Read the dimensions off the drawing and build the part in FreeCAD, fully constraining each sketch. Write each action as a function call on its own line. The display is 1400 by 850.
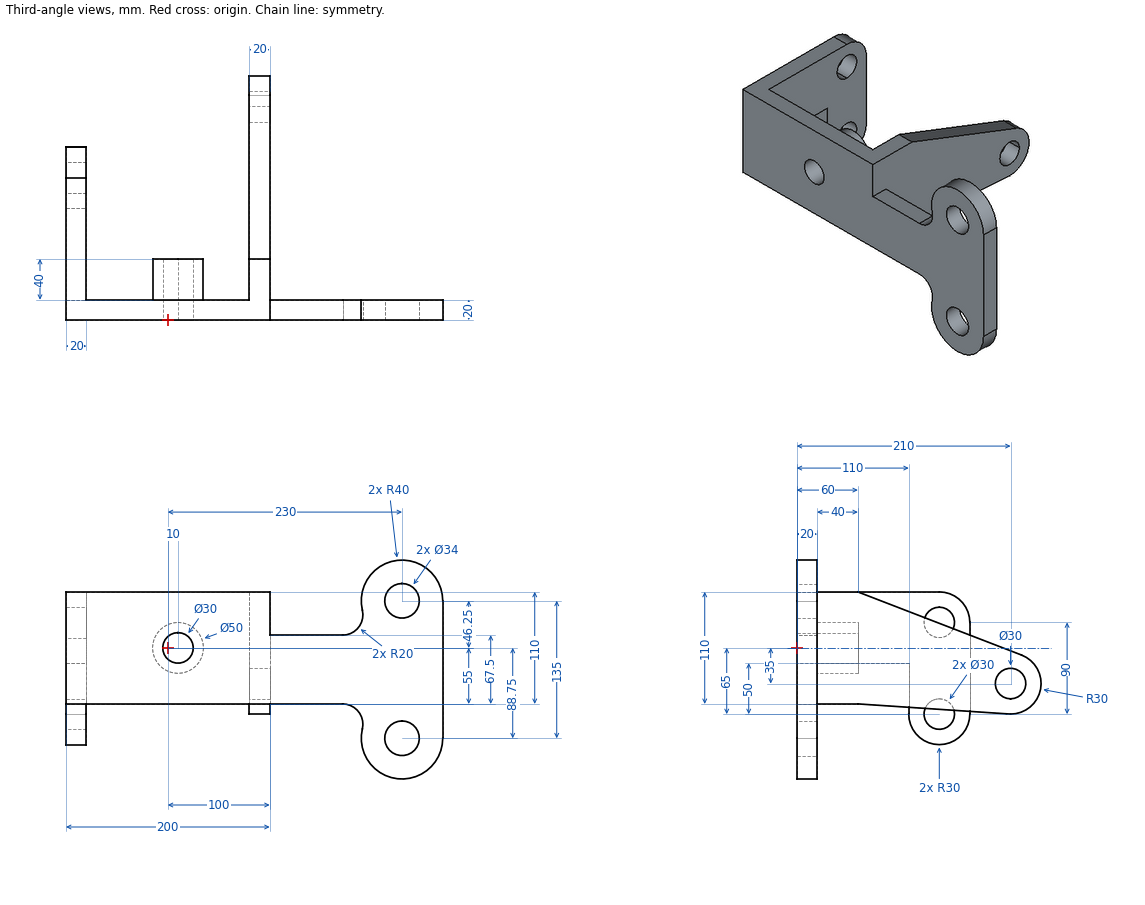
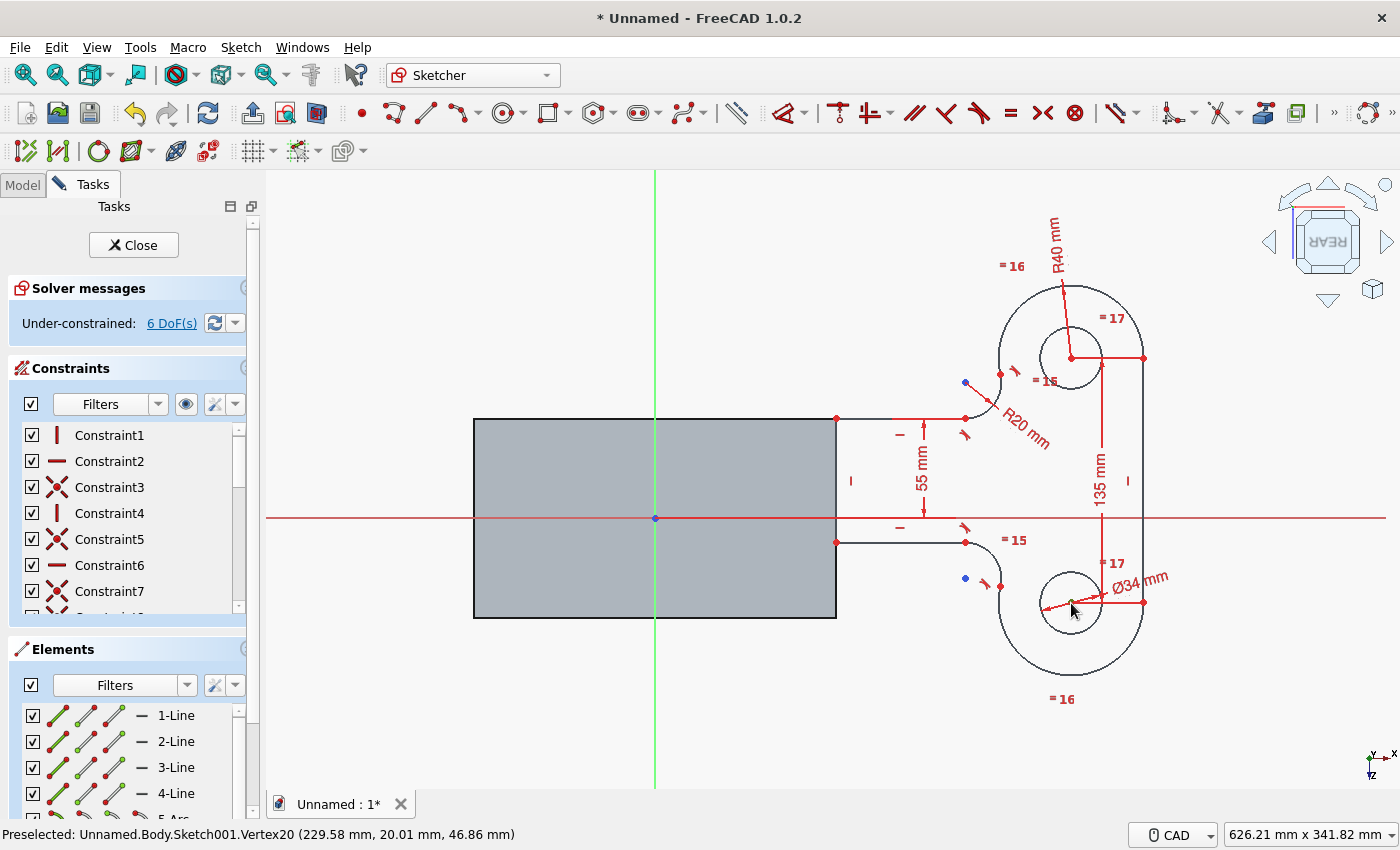
key(l)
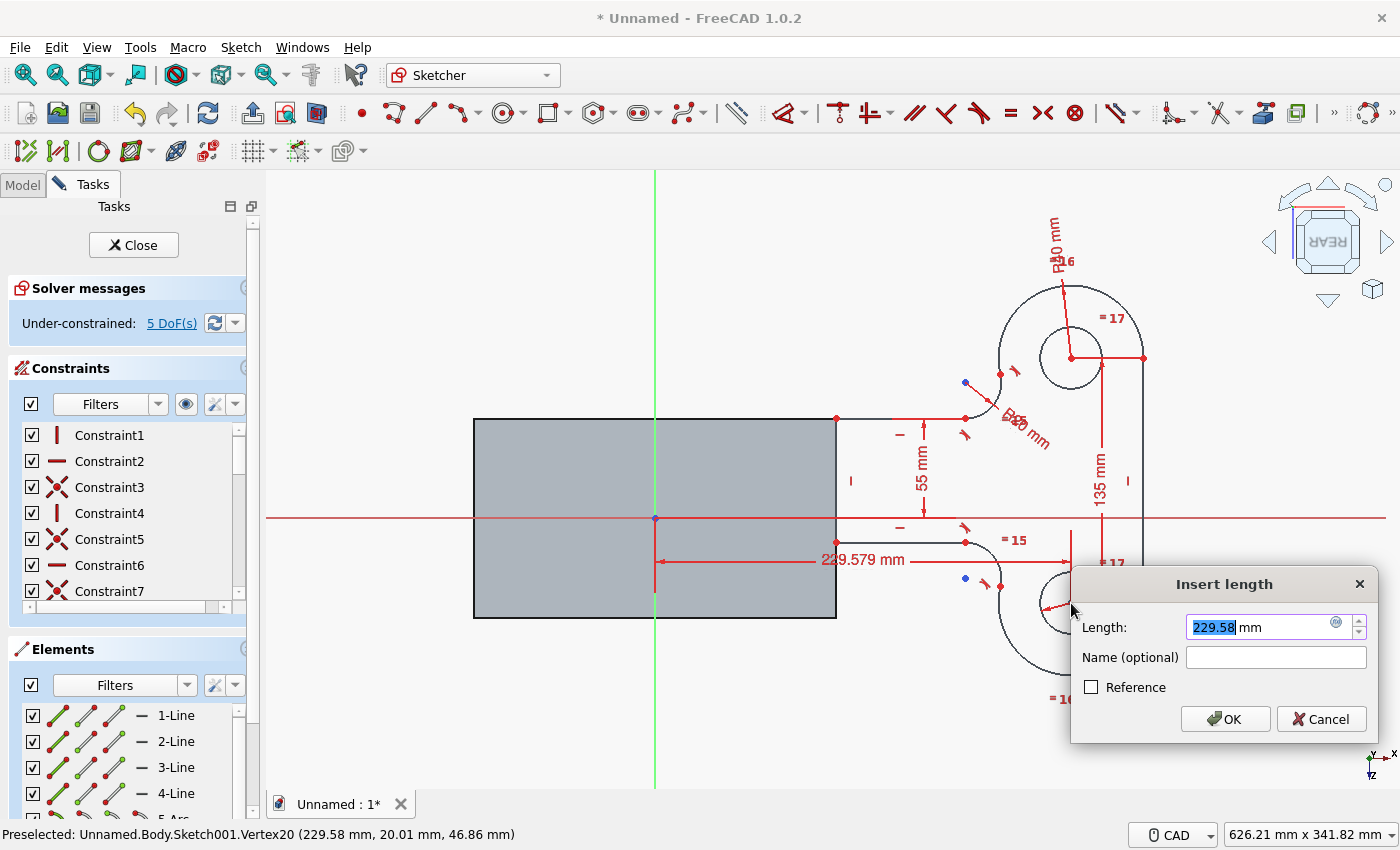
text(230)
key(Return)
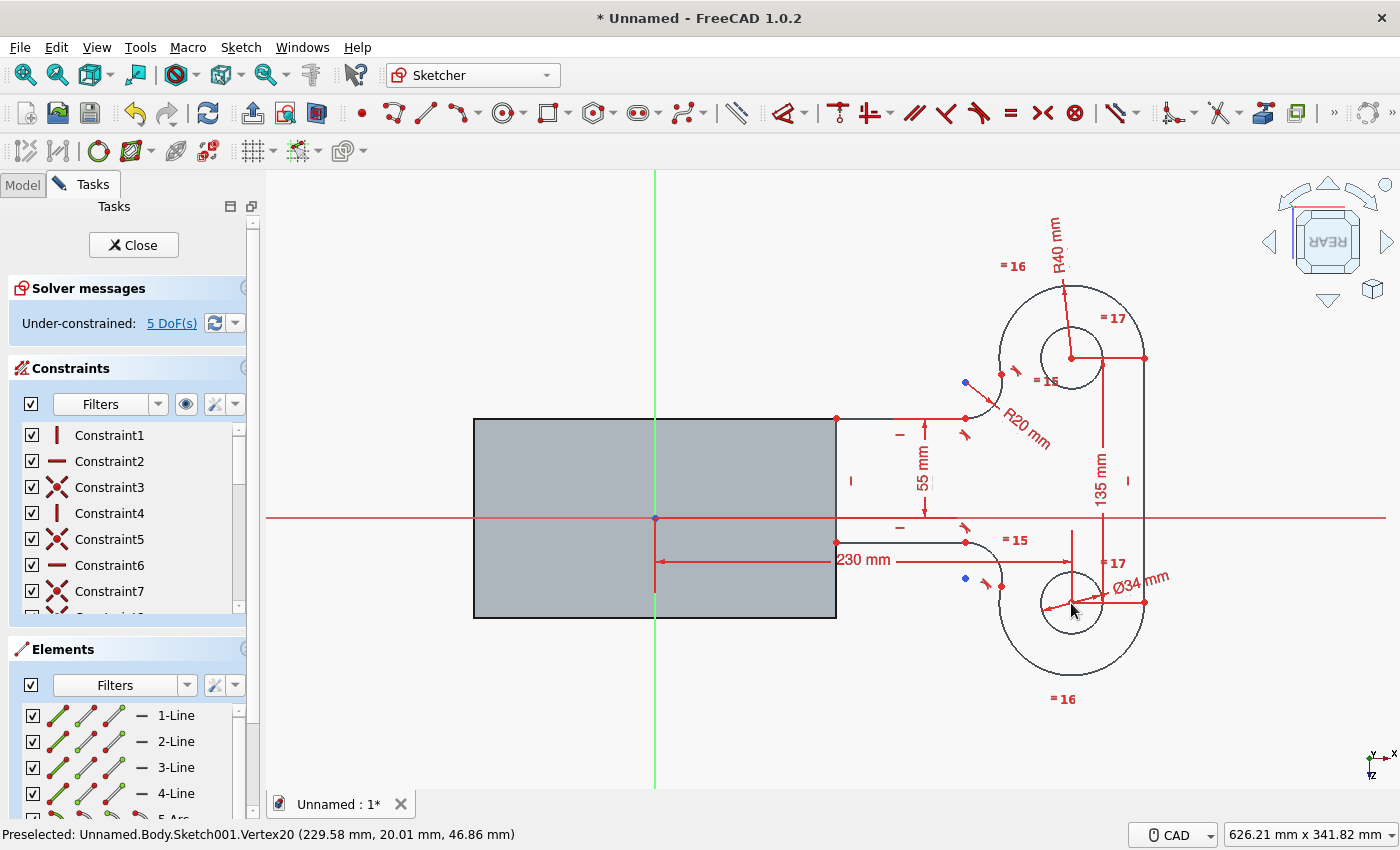
click(836, 456)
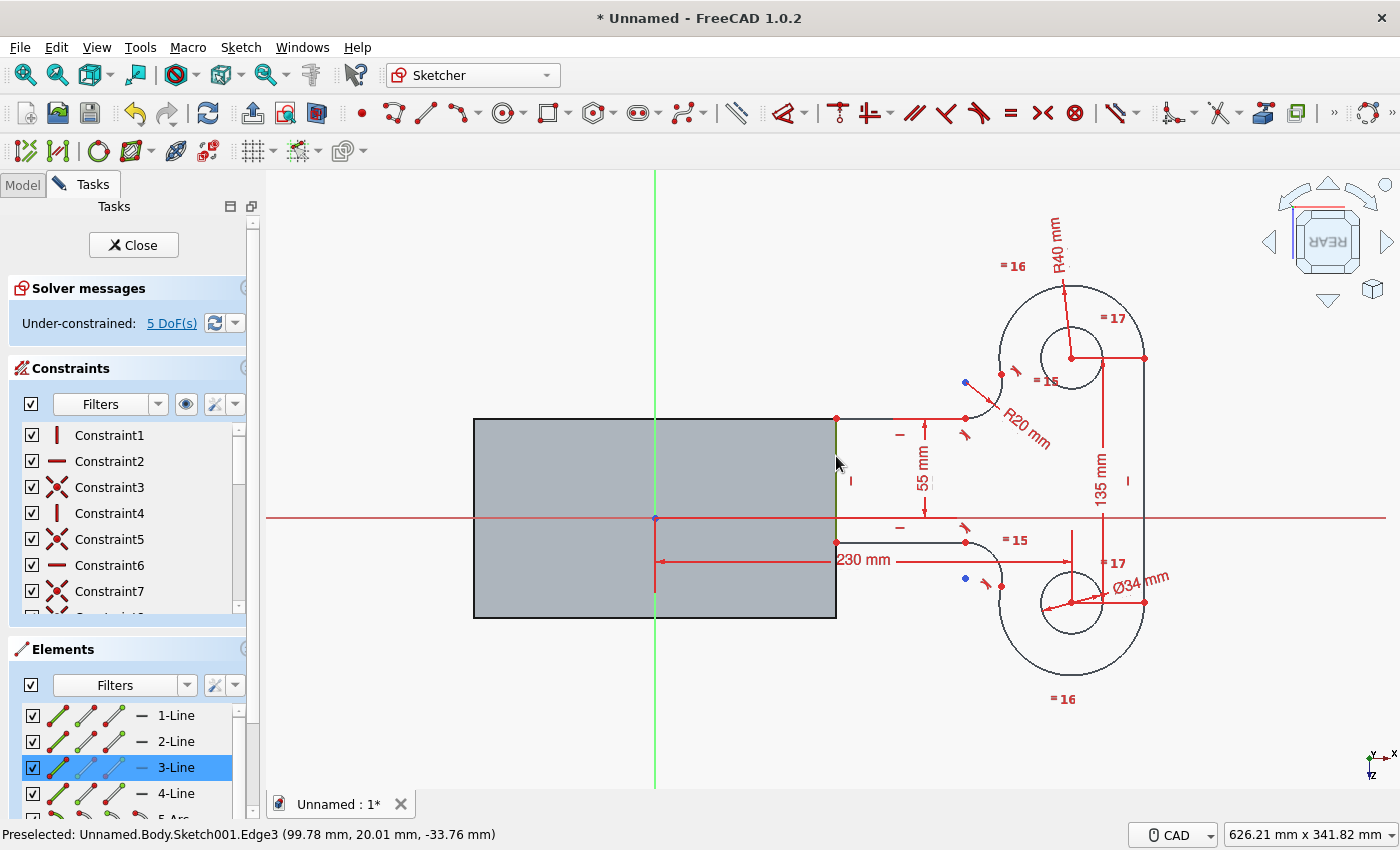
key(i)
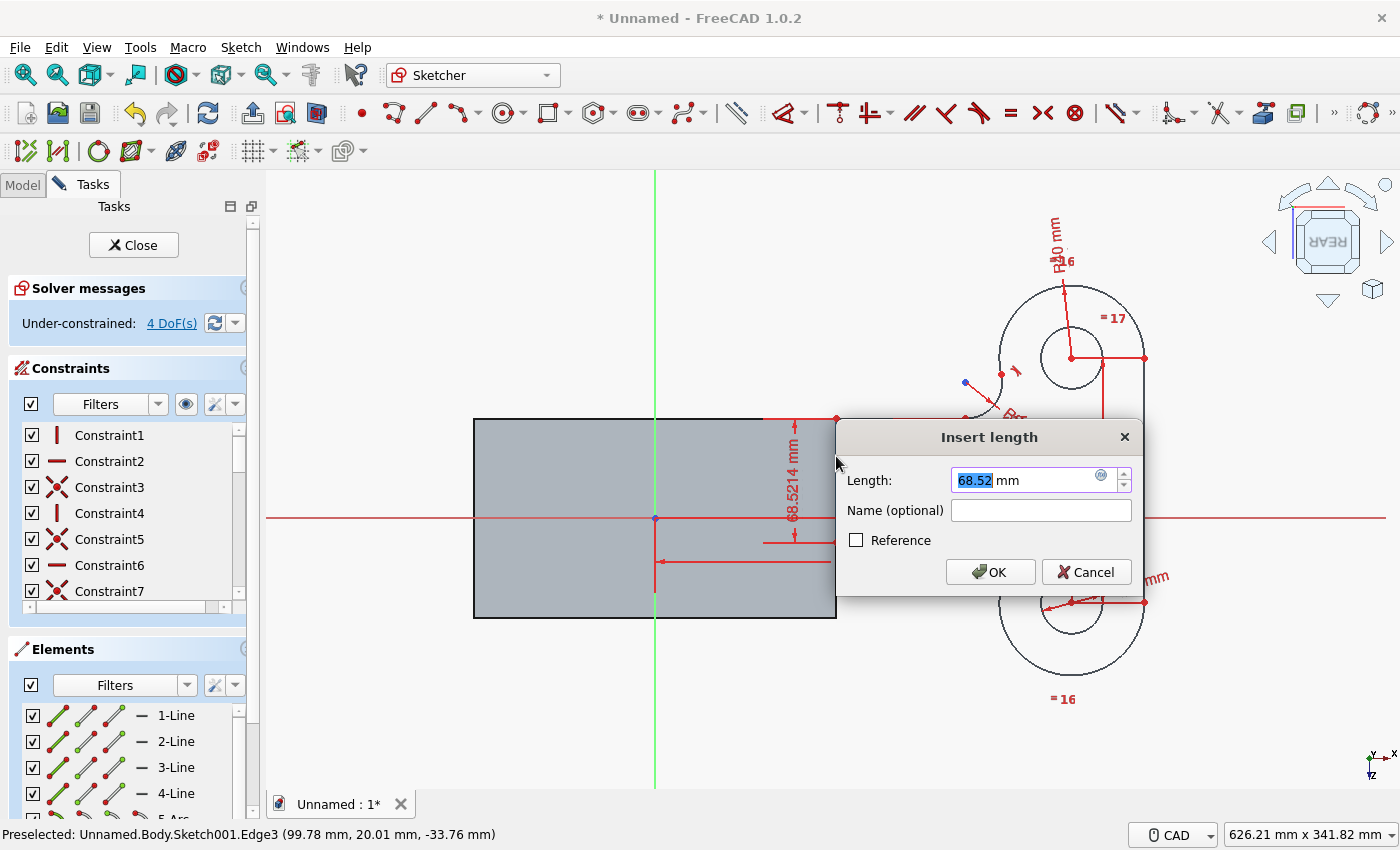
text(67.5)
key(Return)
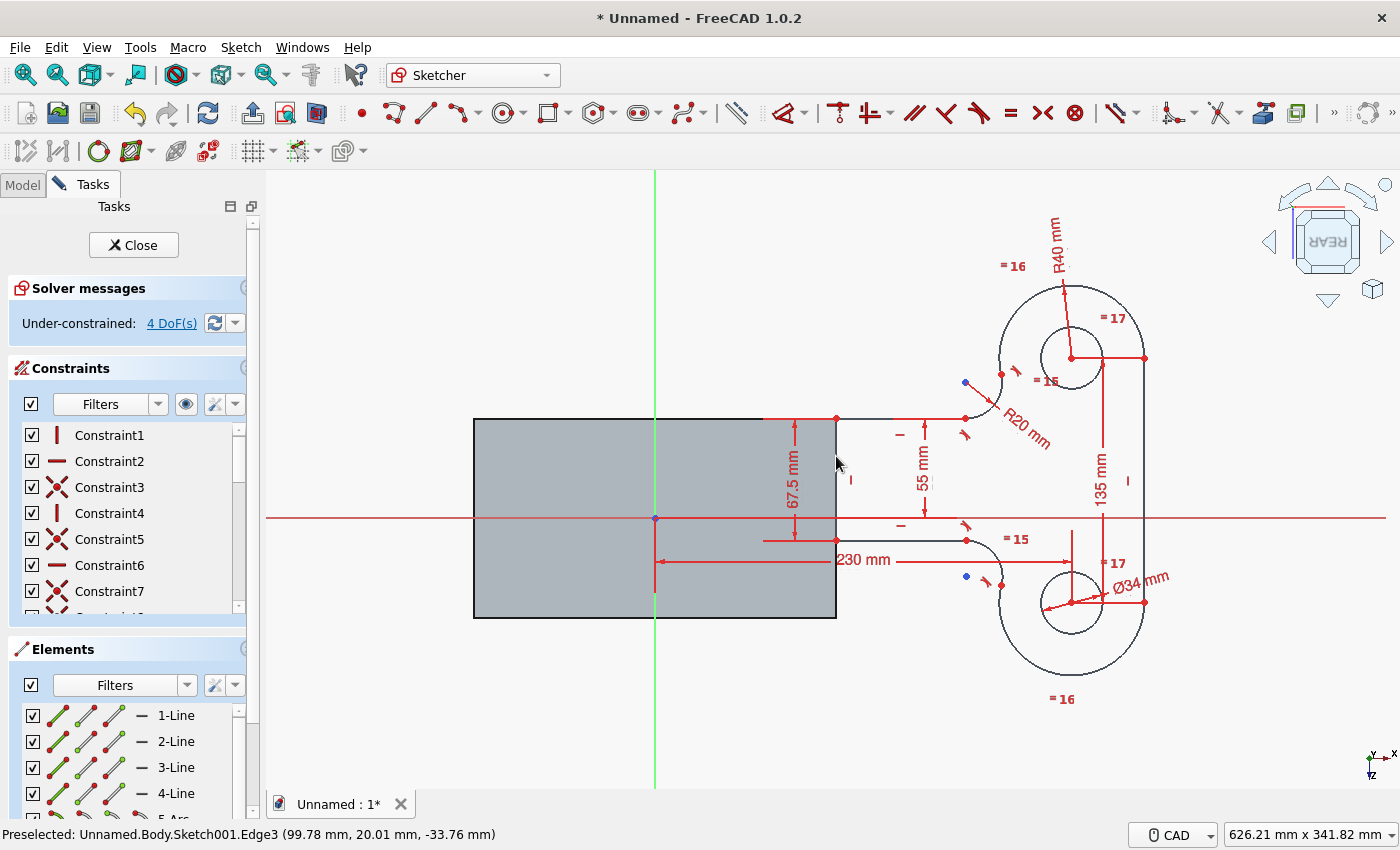
click(836, 419)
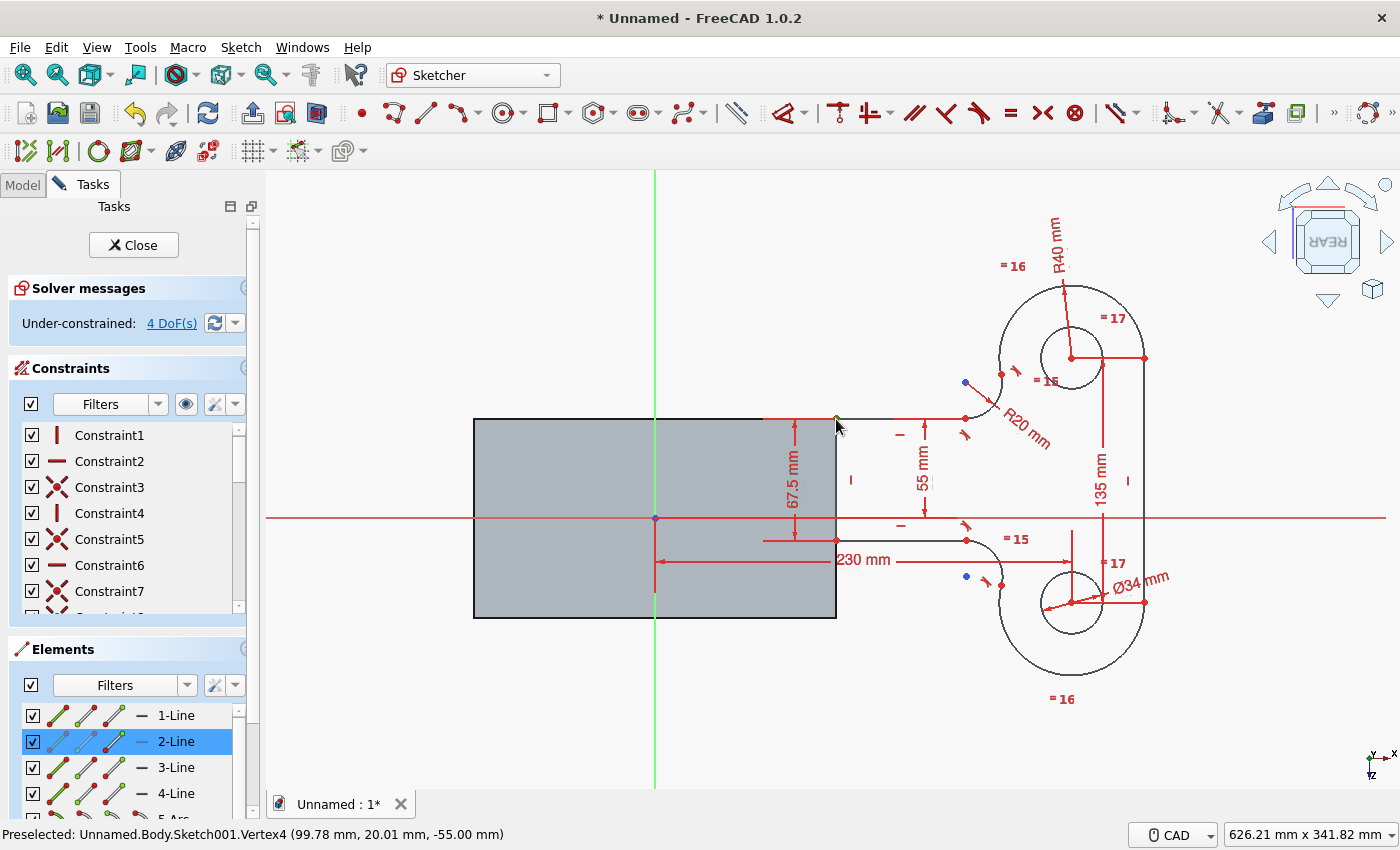
click(806, 114)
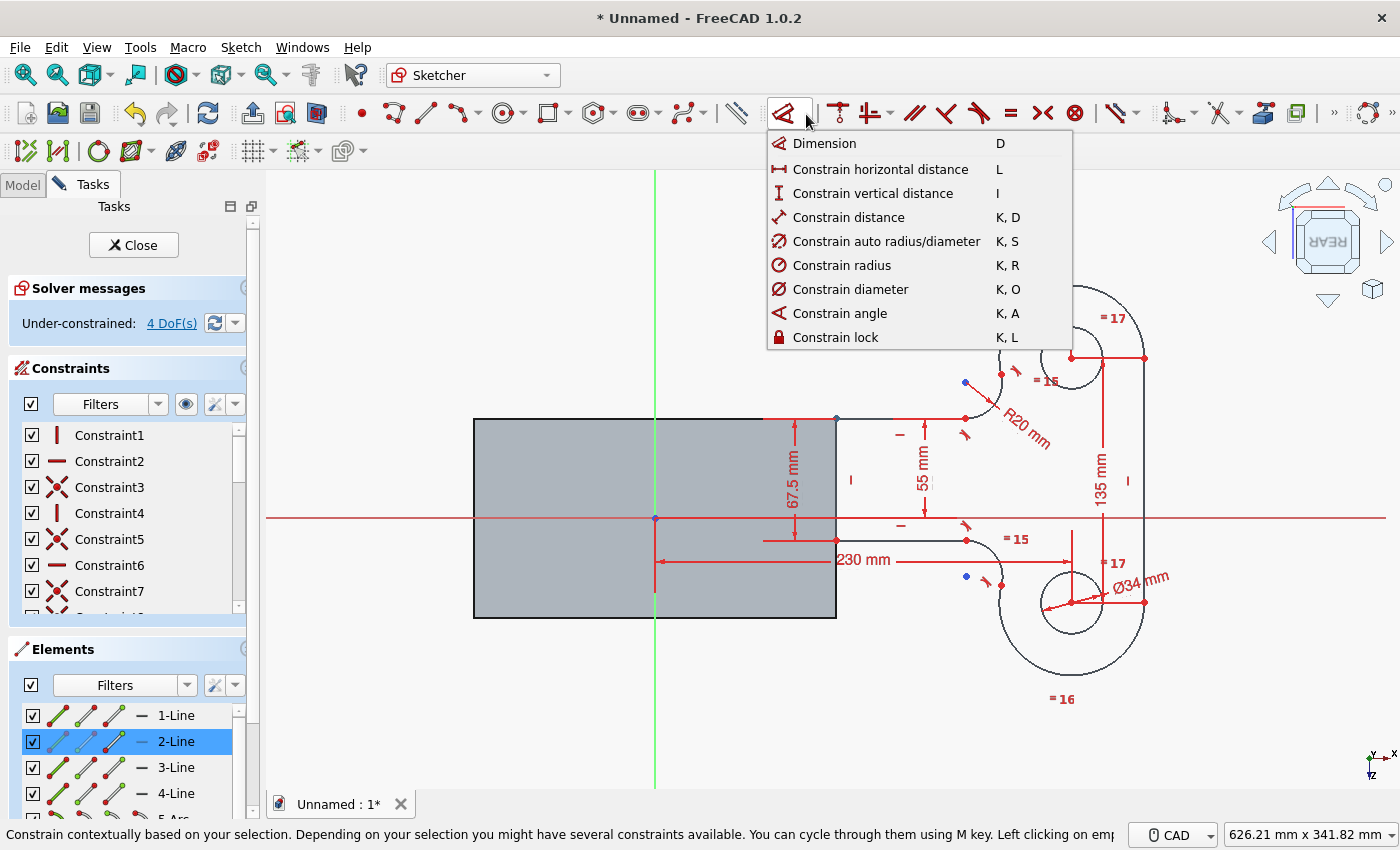
click(920, 169)